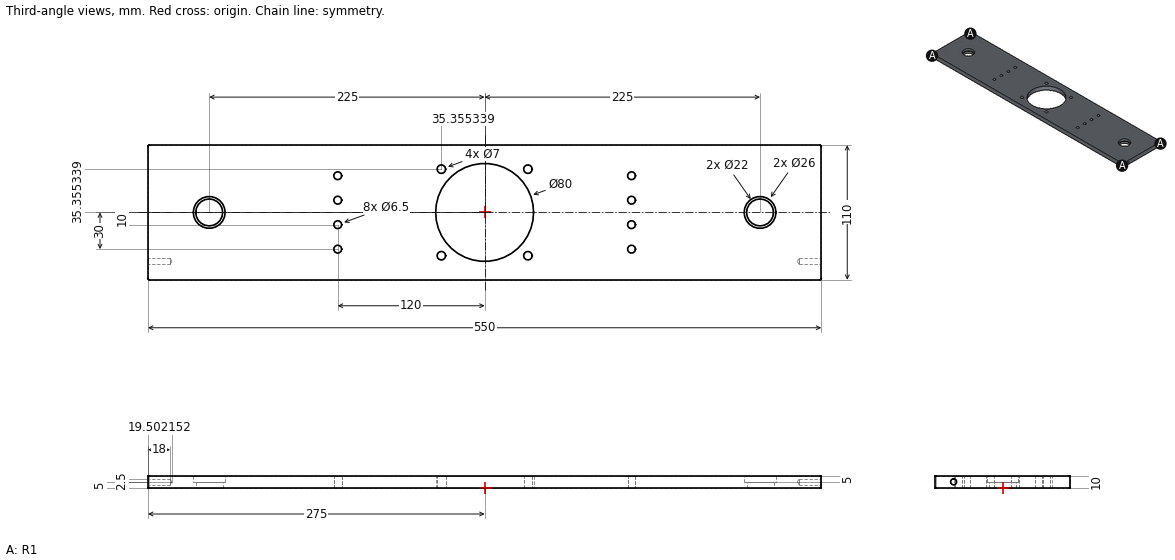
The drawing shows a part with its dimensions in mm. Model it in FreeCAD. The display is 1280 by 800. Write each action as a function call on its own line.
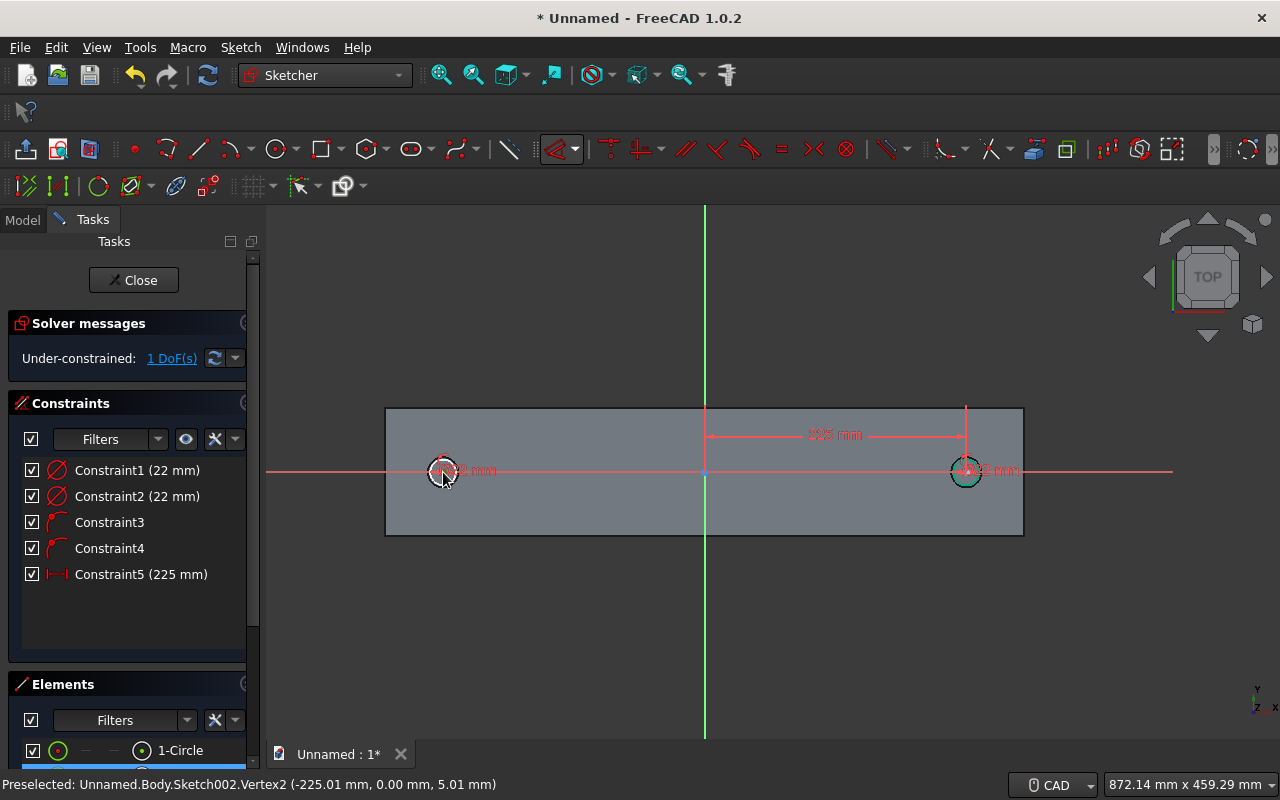
key(l)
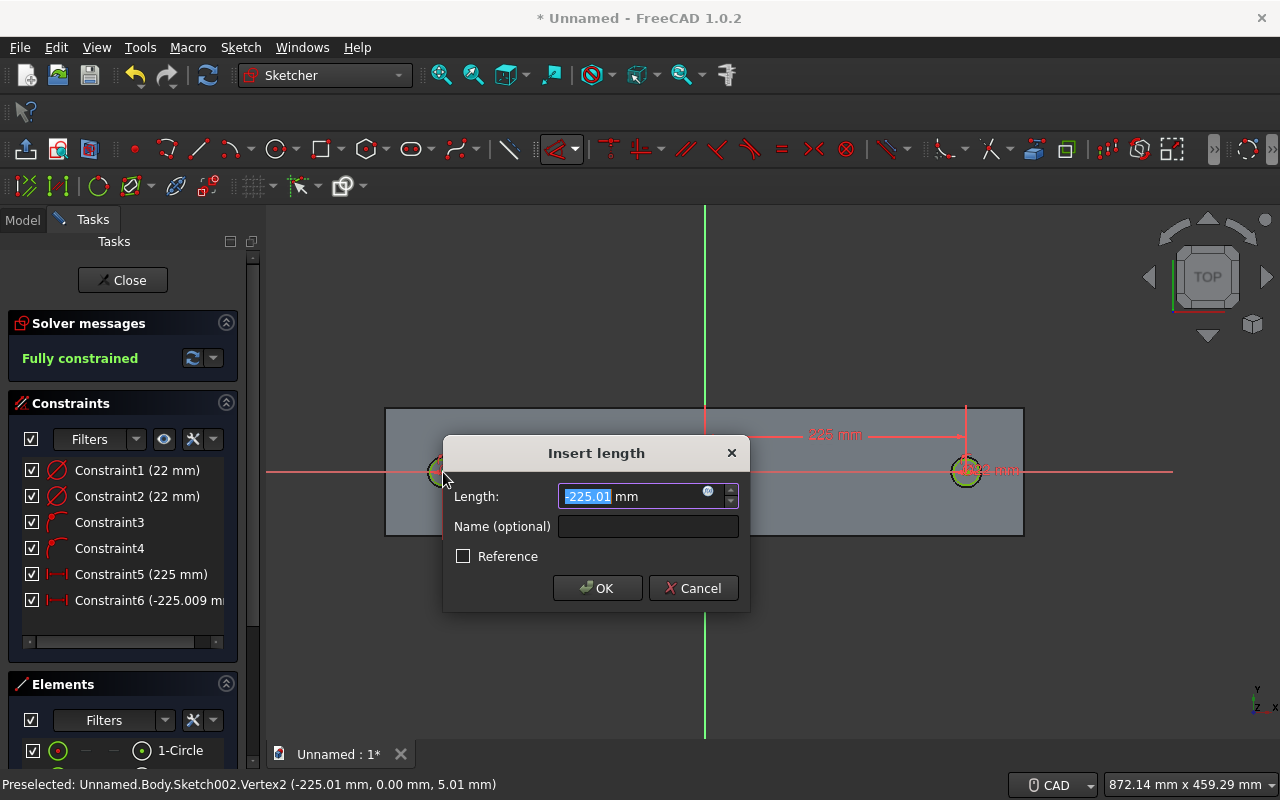
text(-225)
key(Return)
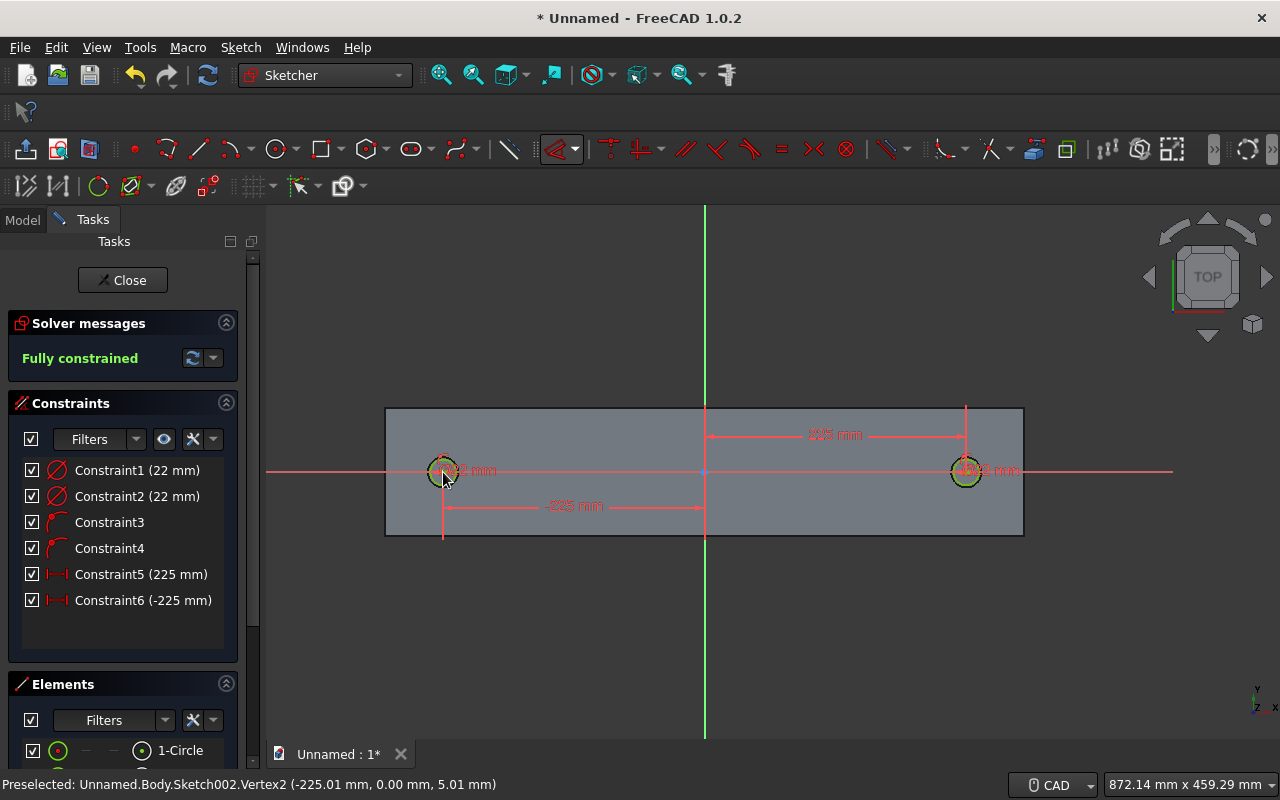
click(123, 280)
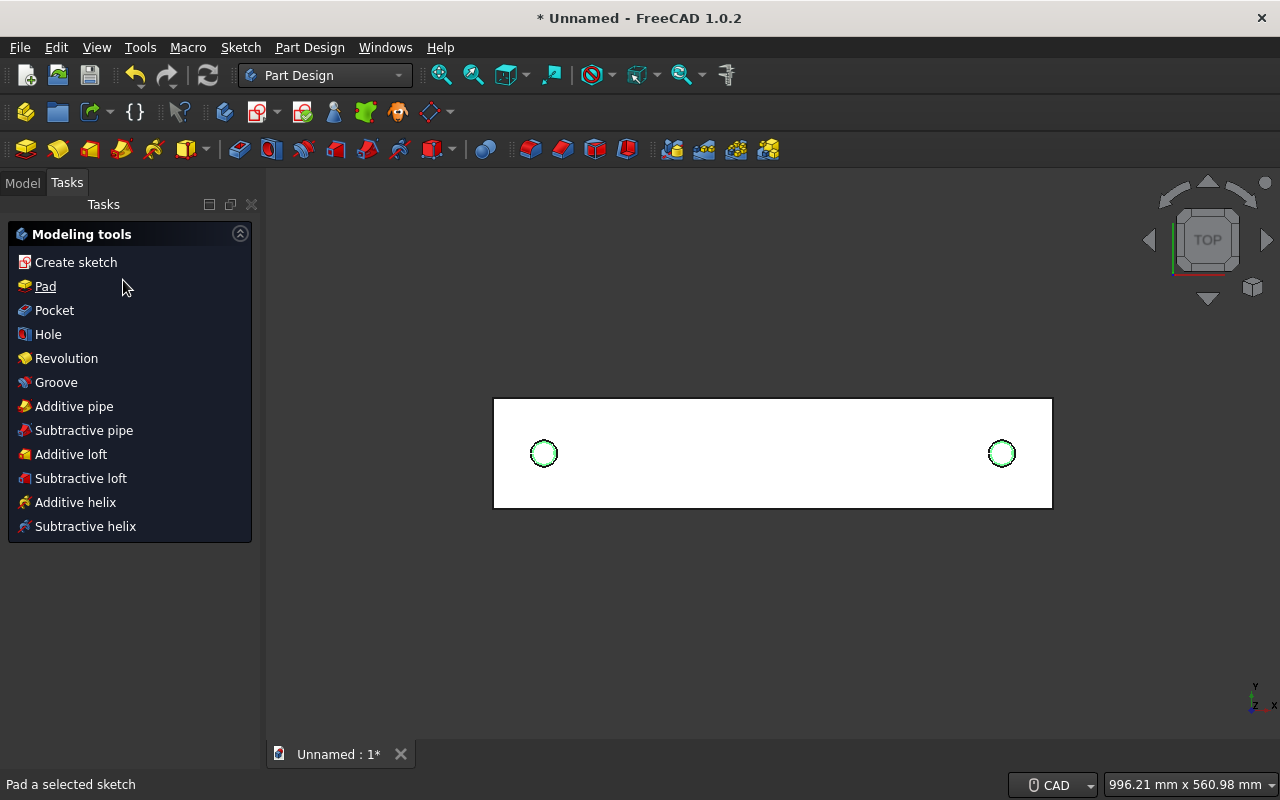
click(240, 150)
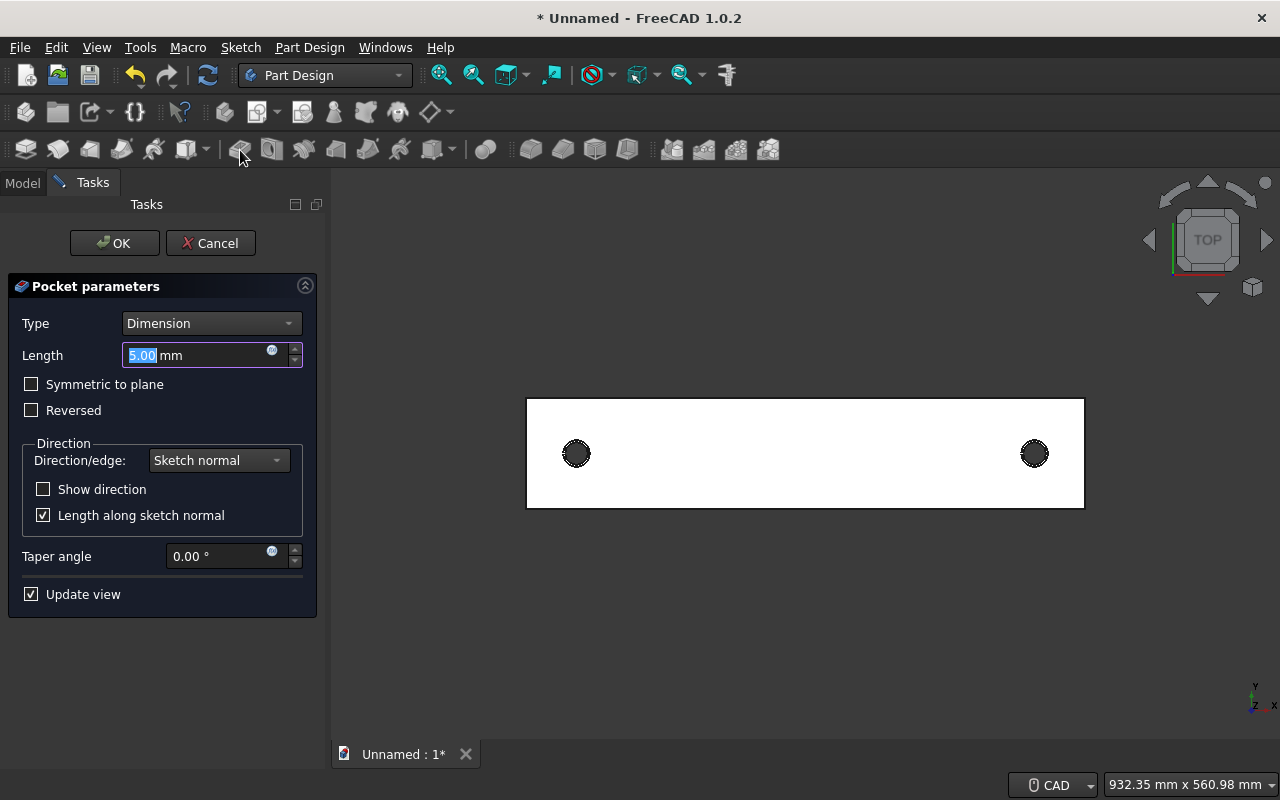
click(212, 324)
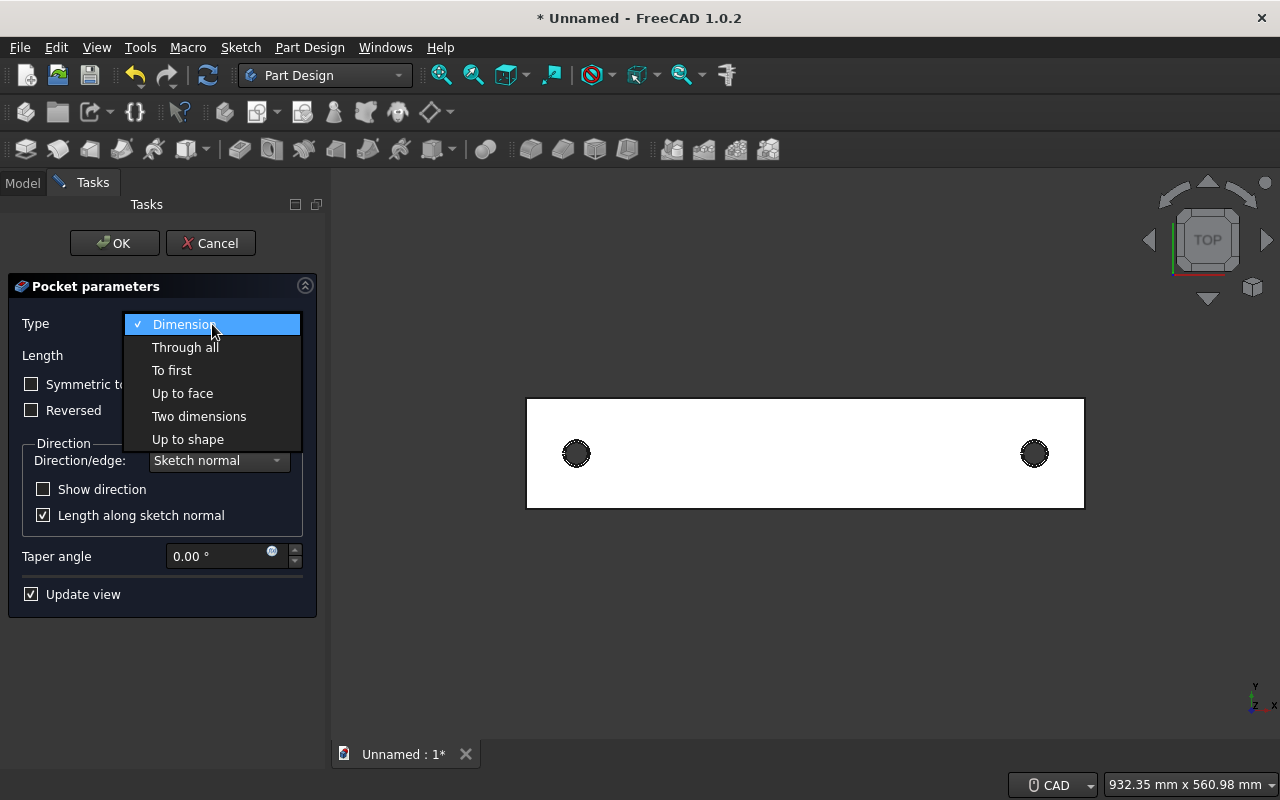
click(212, 348)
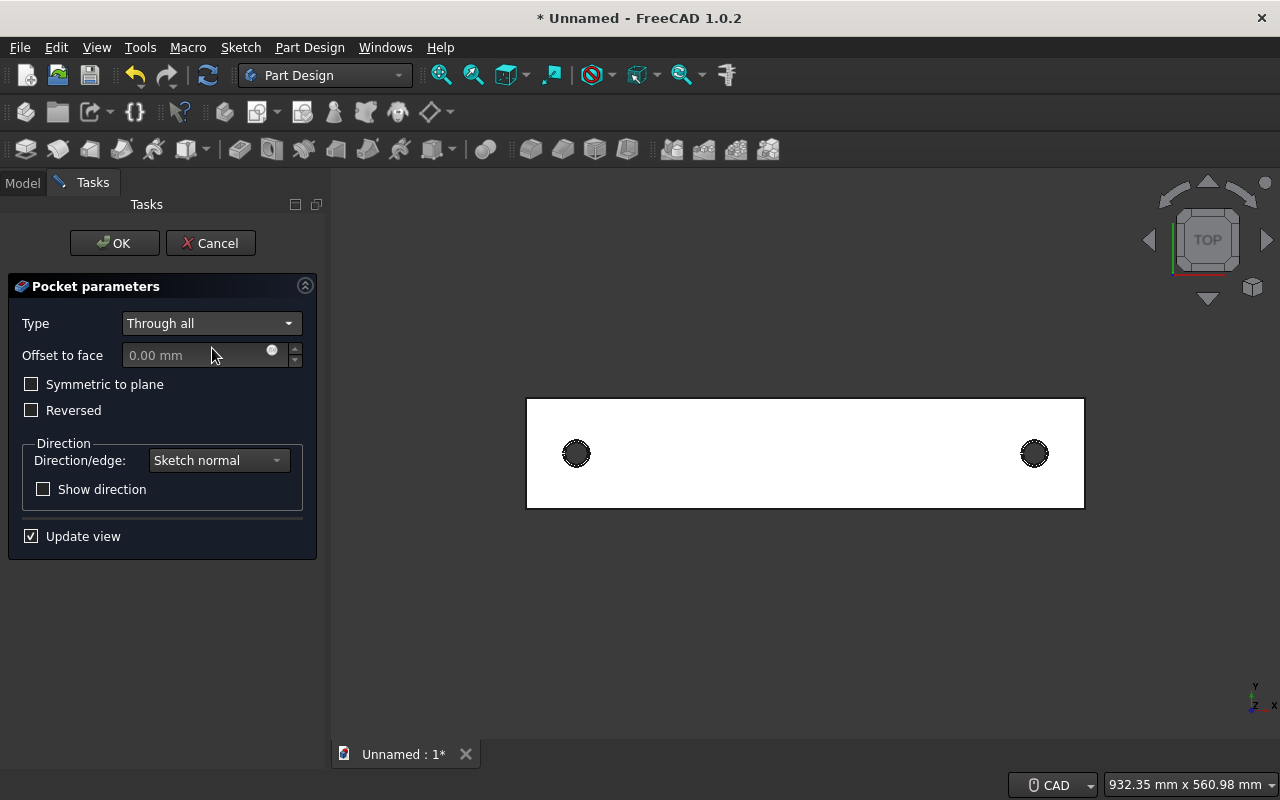
click(115, 243)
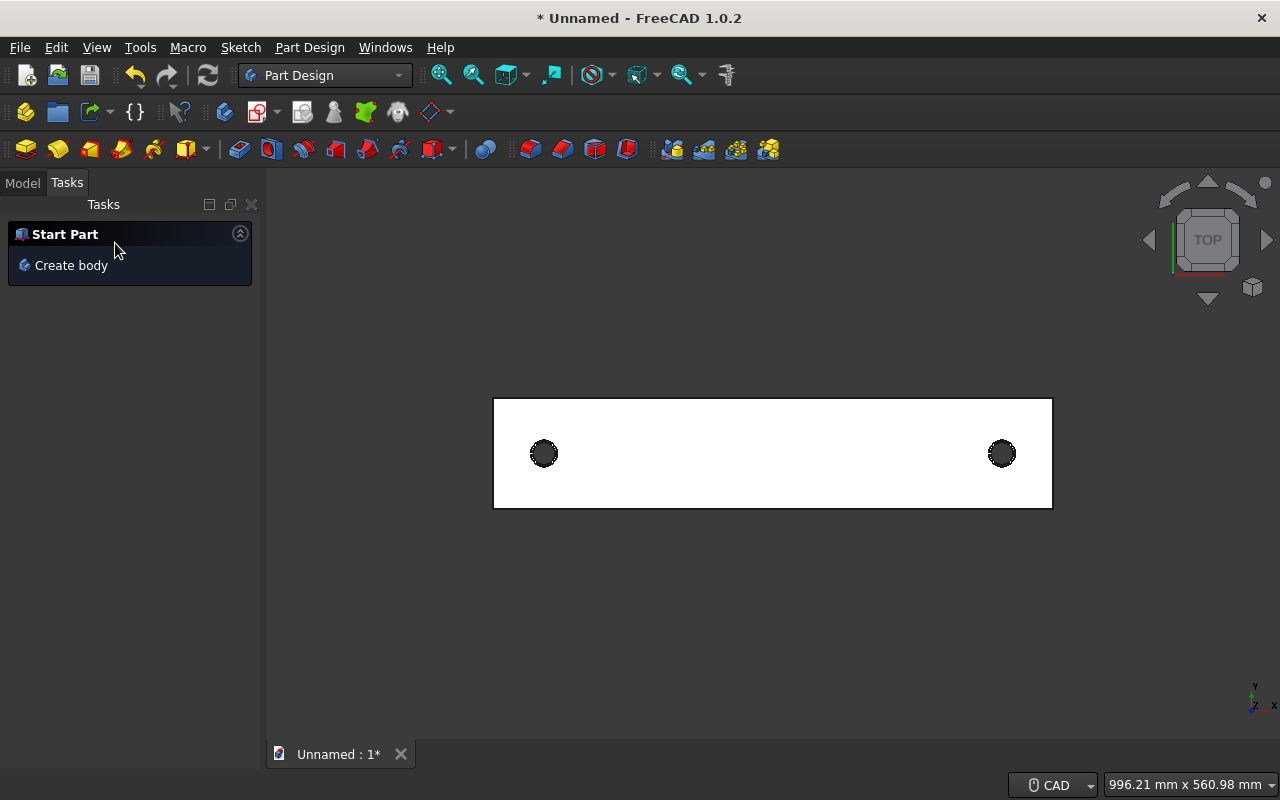
click(853, 452)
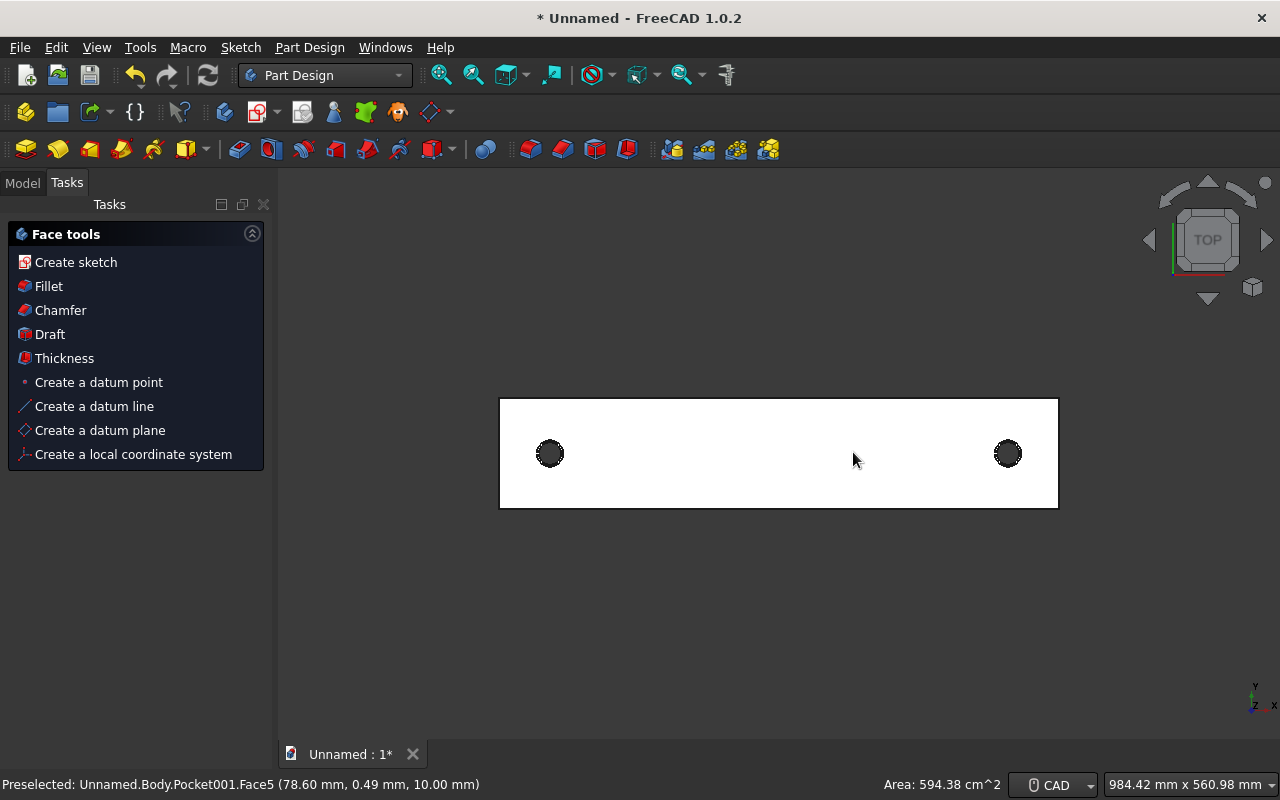
click(258, 112)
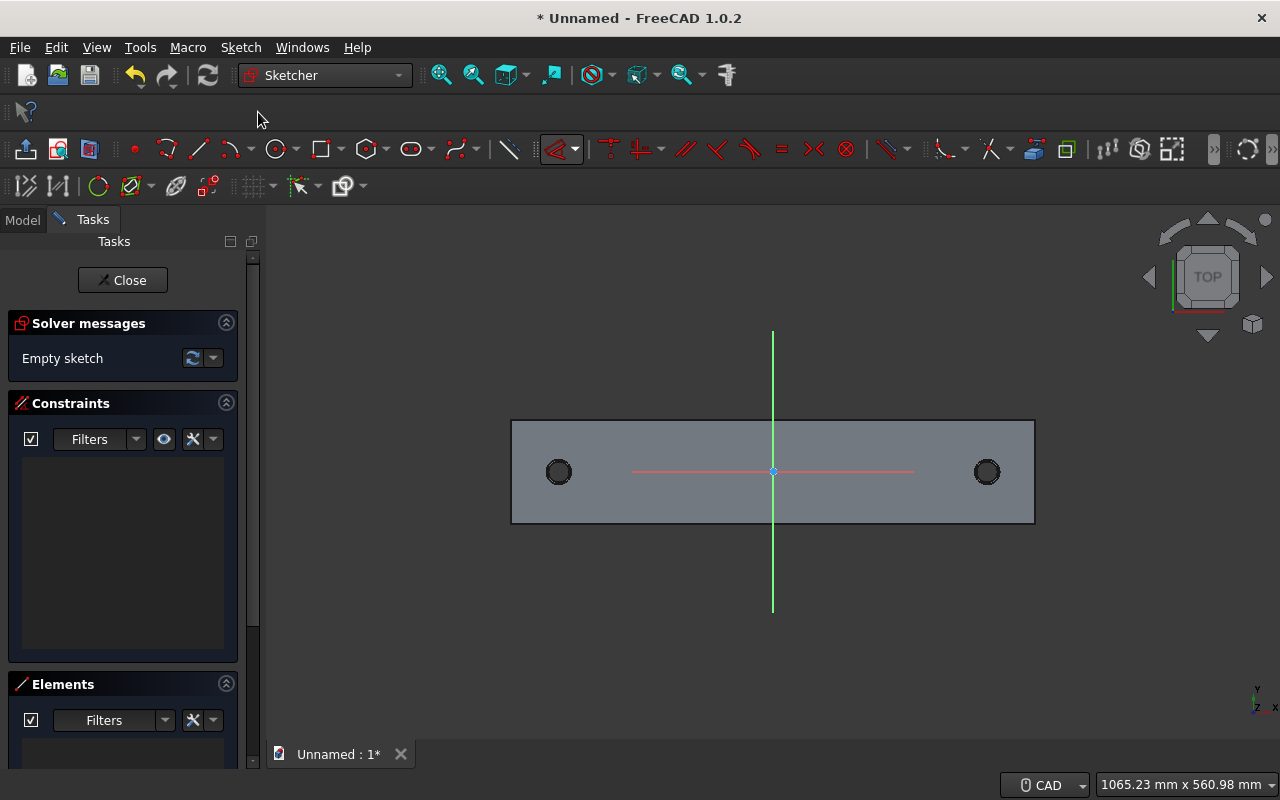
scroll(795, 472, up, 7)